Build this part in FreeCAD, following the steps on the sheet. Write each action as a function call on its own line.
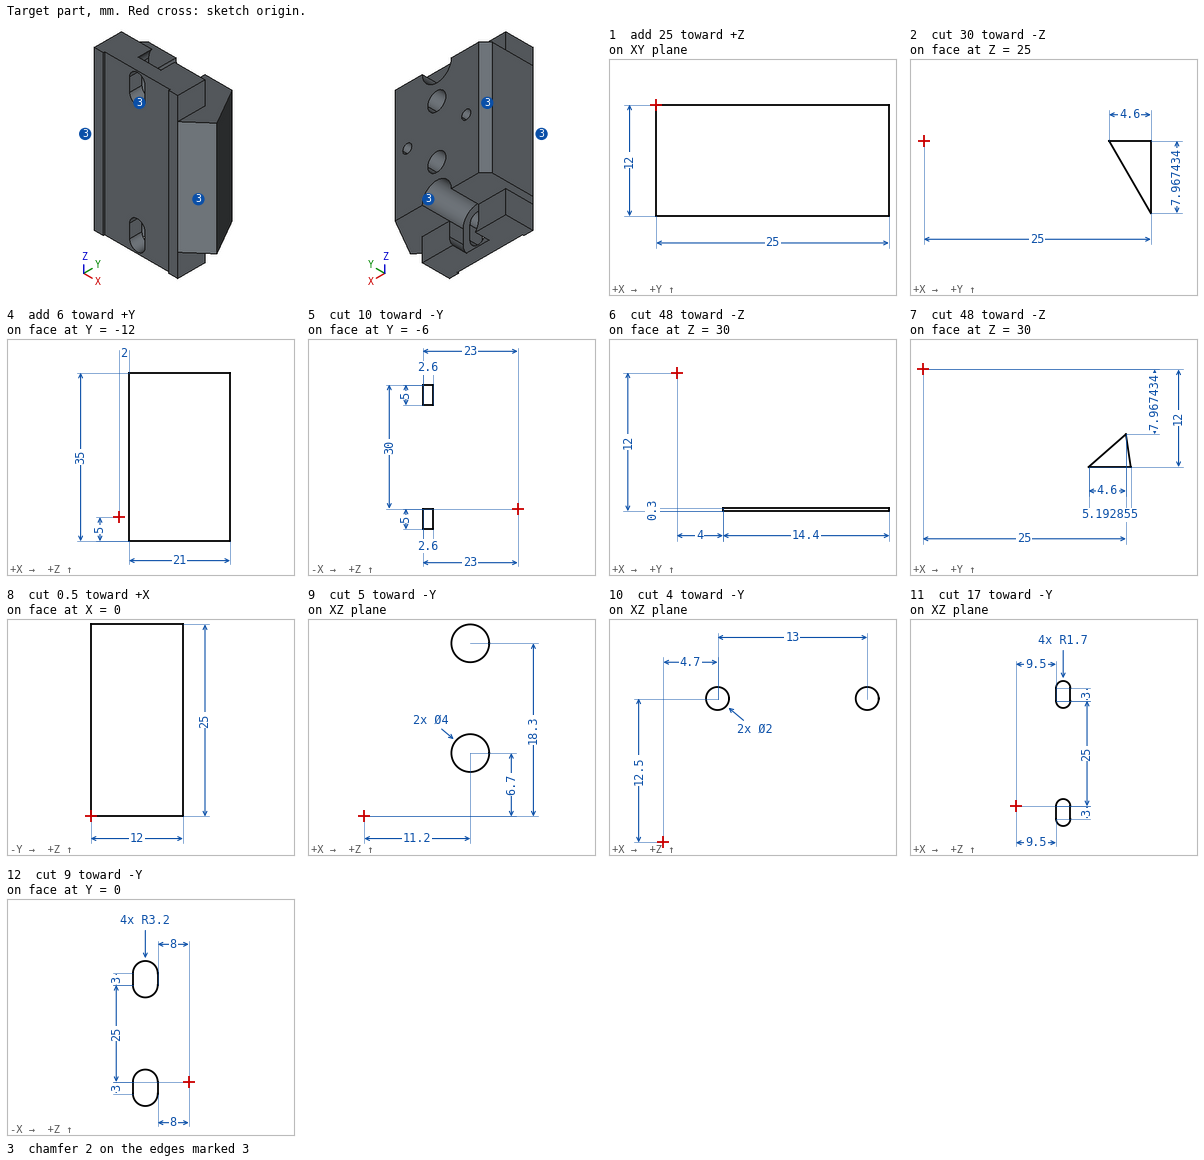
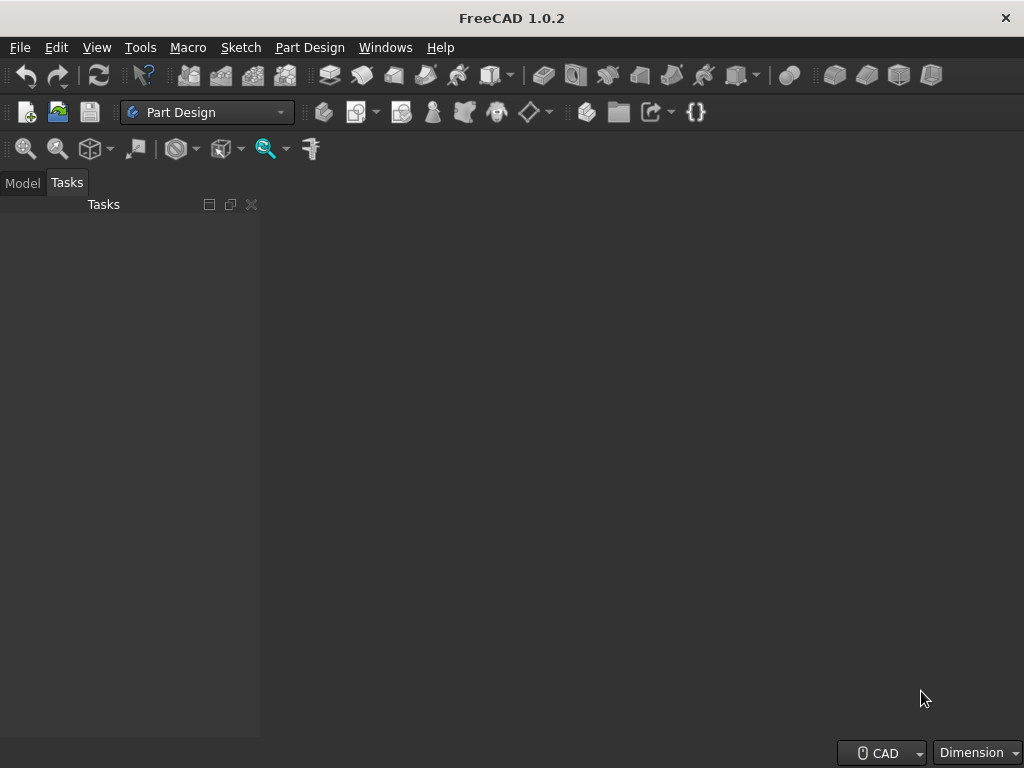
key(ctrl+n)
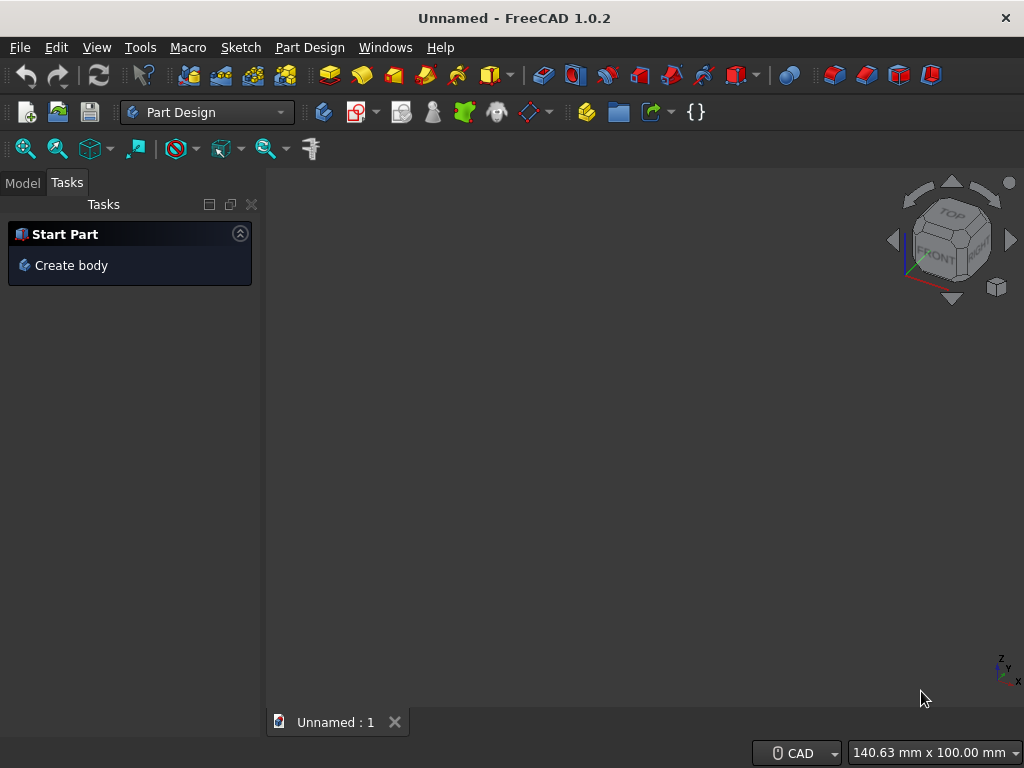
click(356, 112)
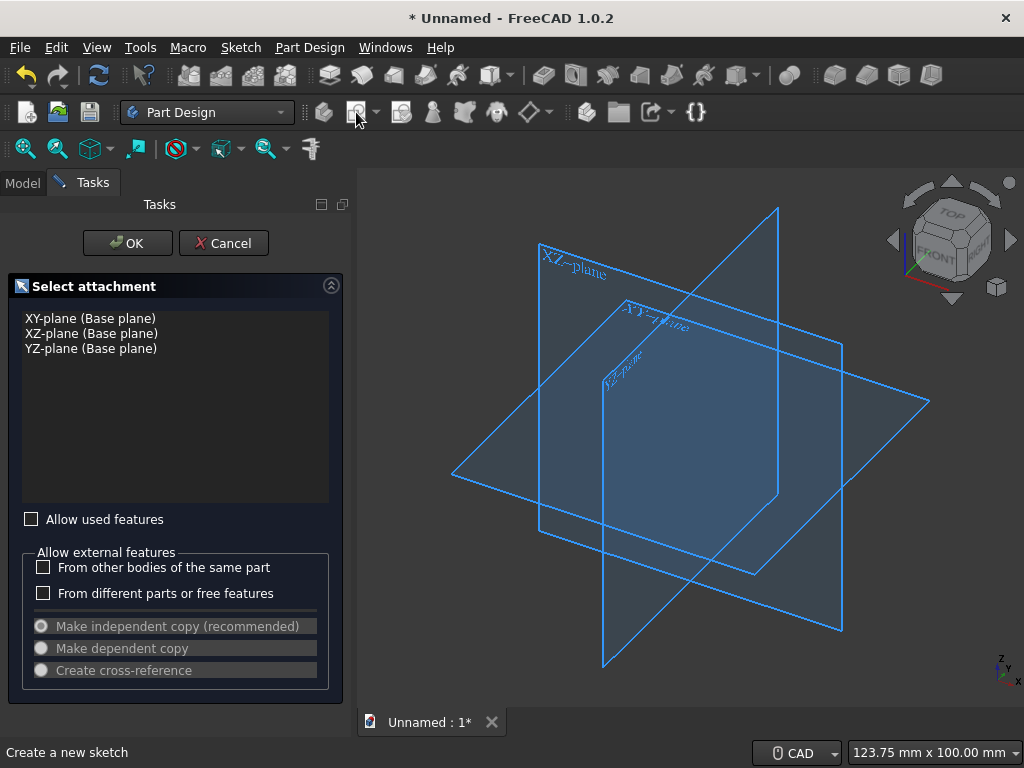
click(82, 318)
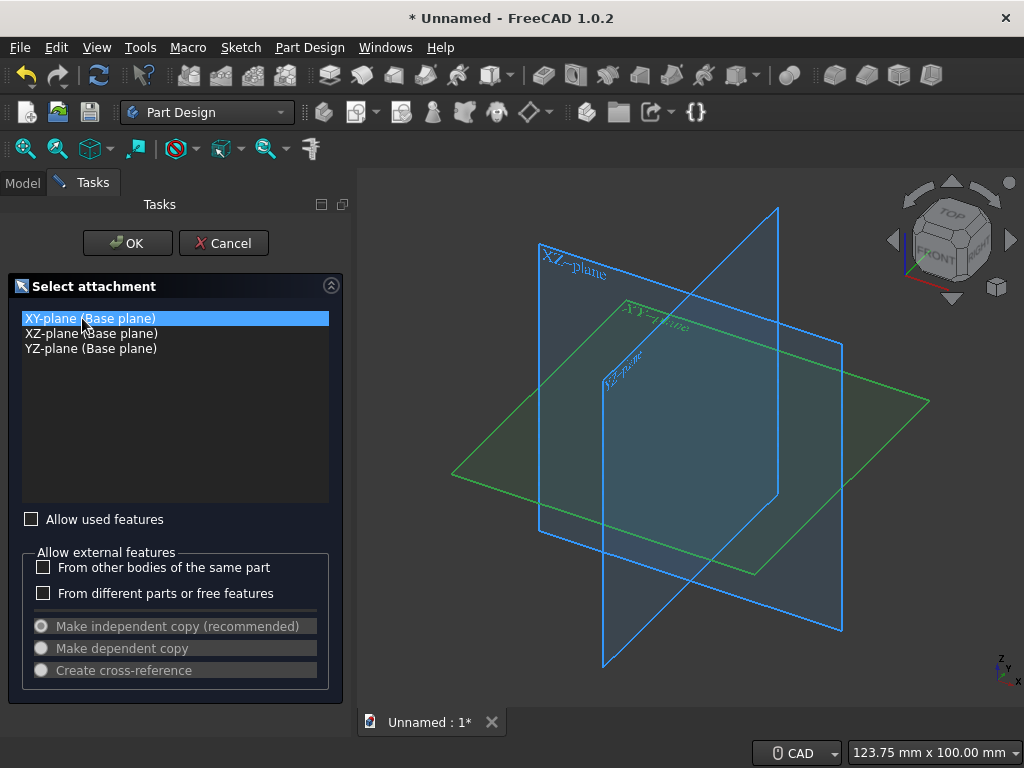
click(128, 243)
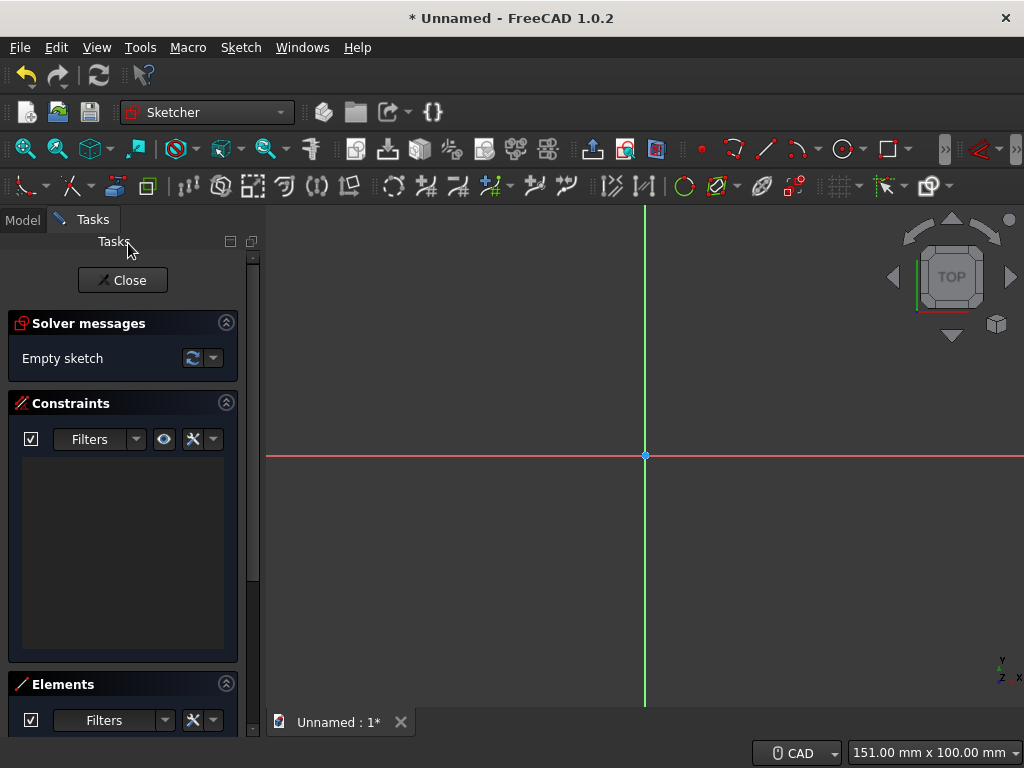
scroll(764, 499, up, 6)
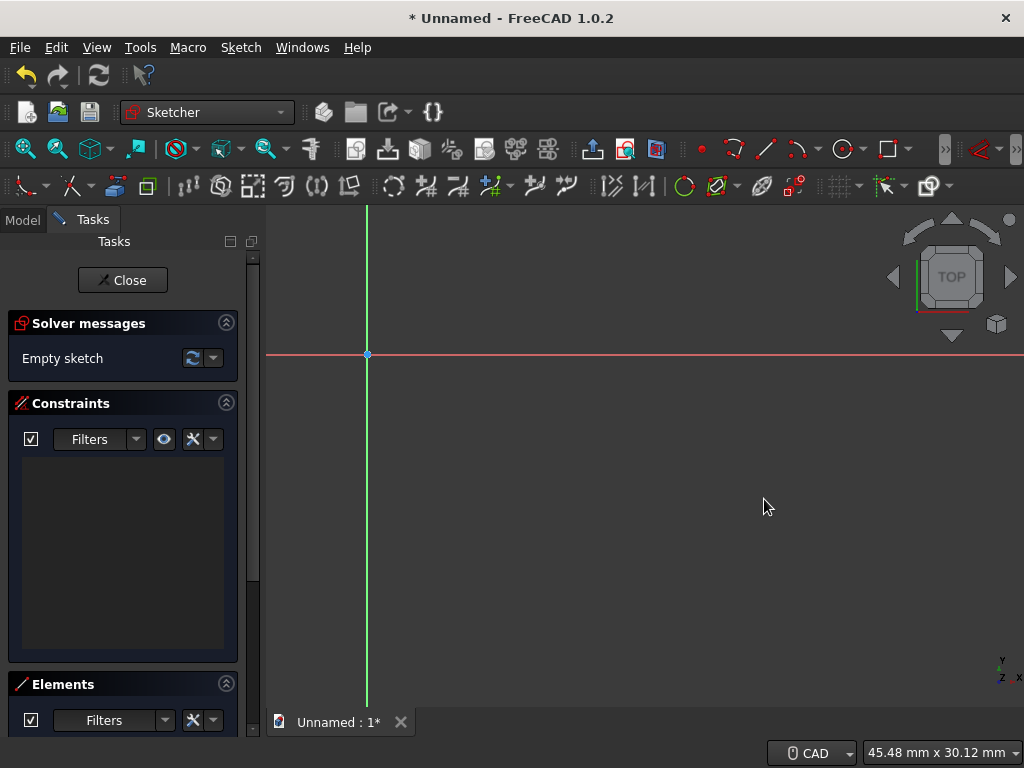
click(888, 150)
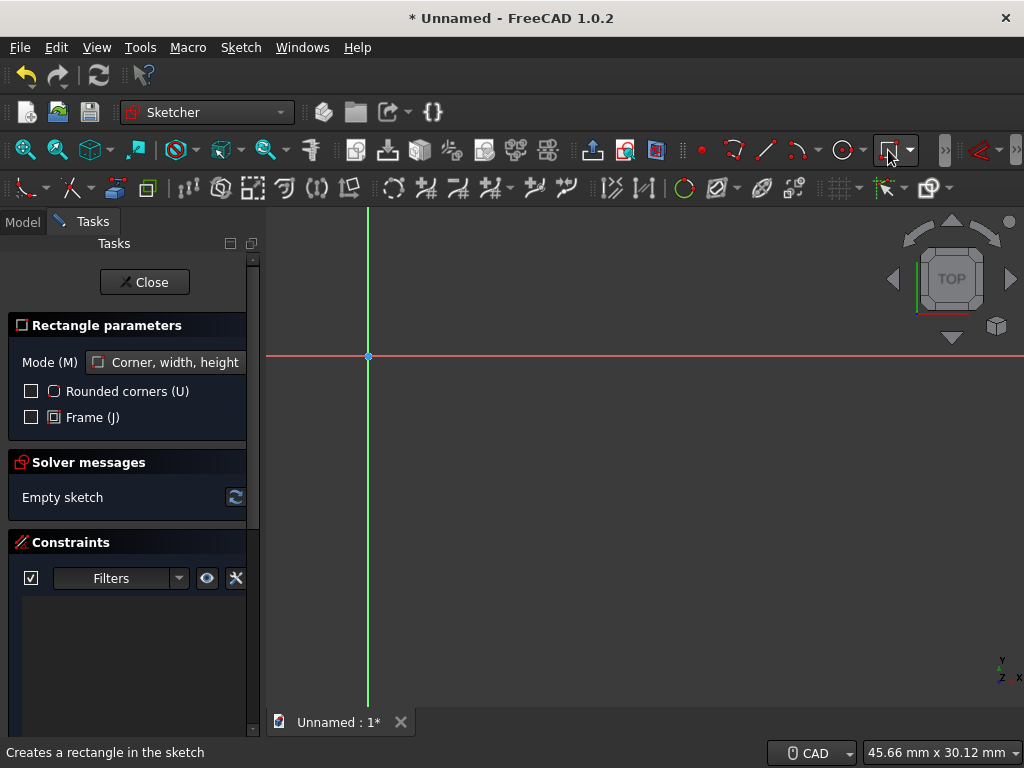
click(368, 356)
click(784, 555)
key(Escape)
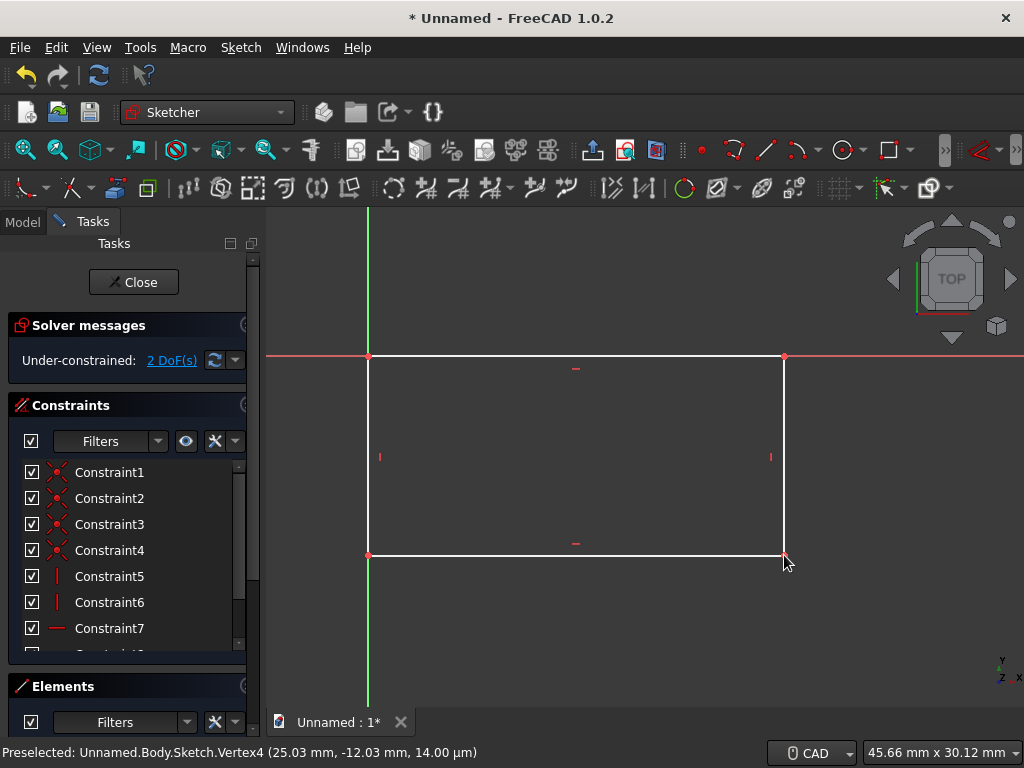
click(368, 416)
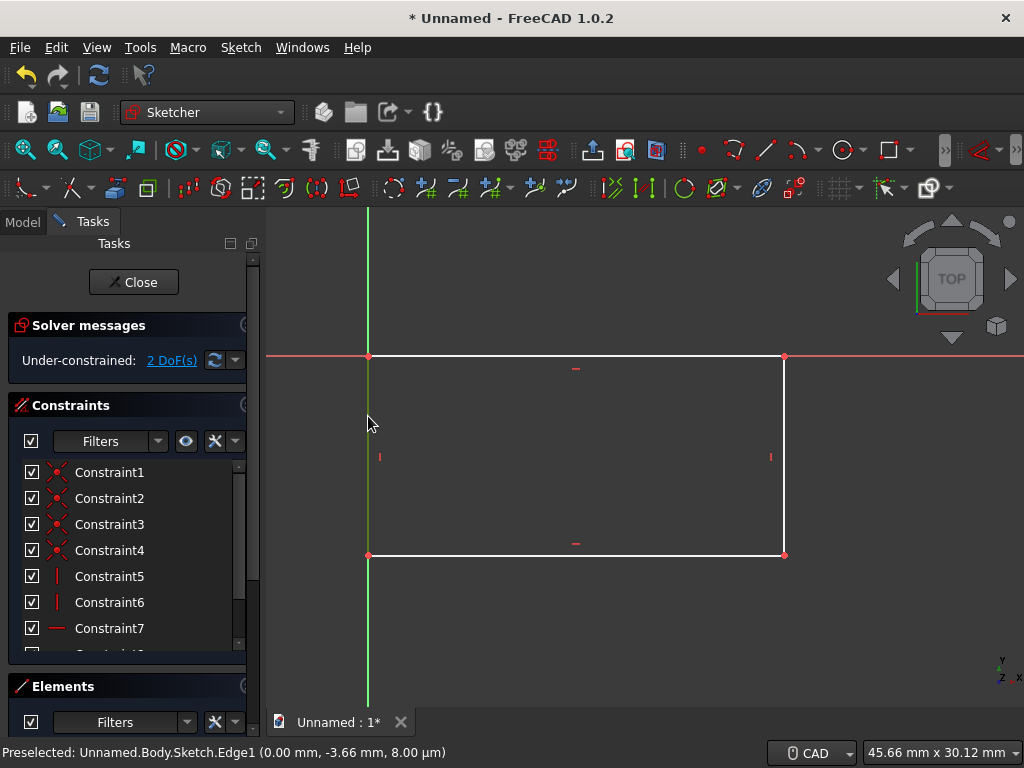
click(1002, 150)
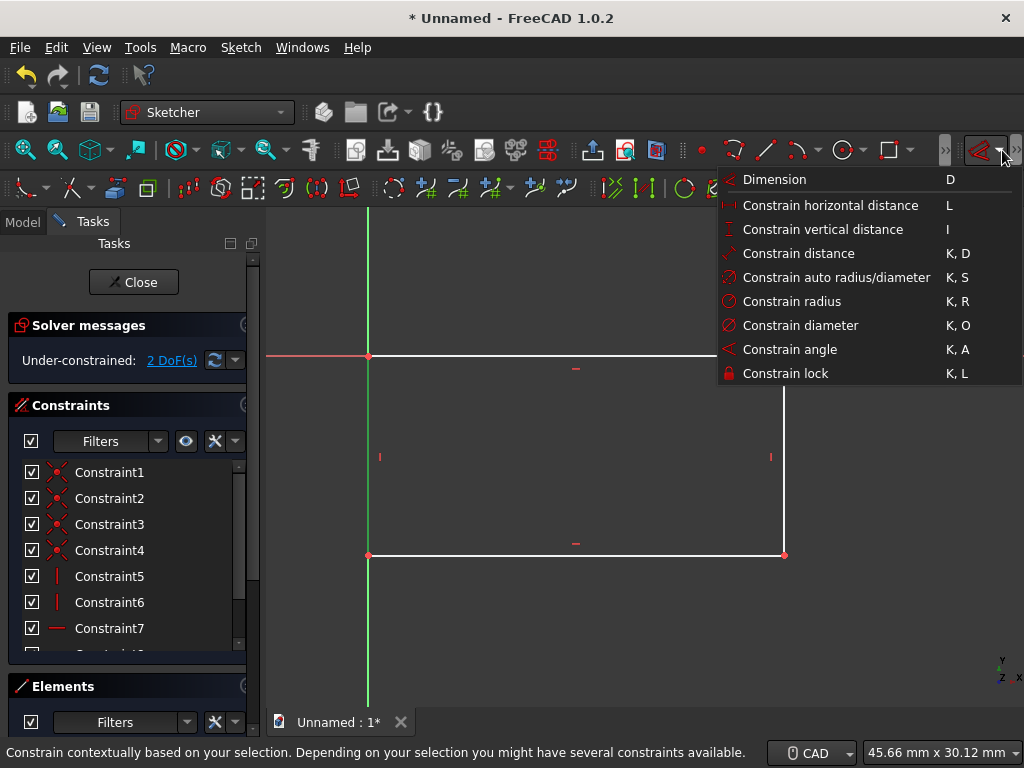
click(870, 229)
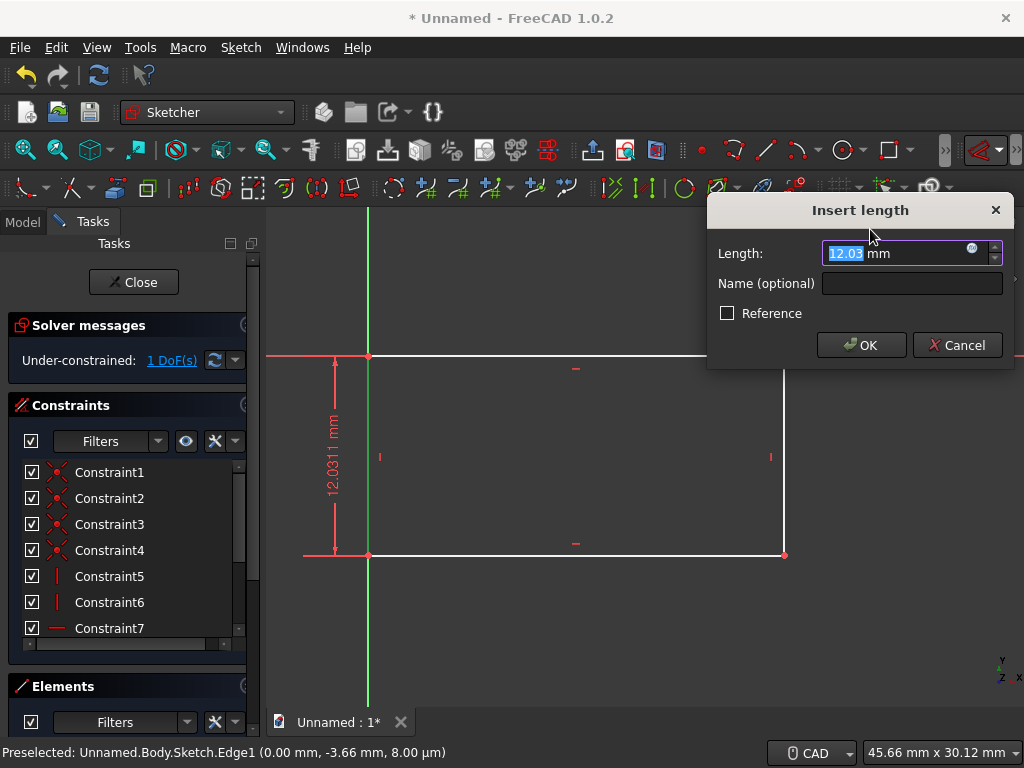
text(12)
key(Return)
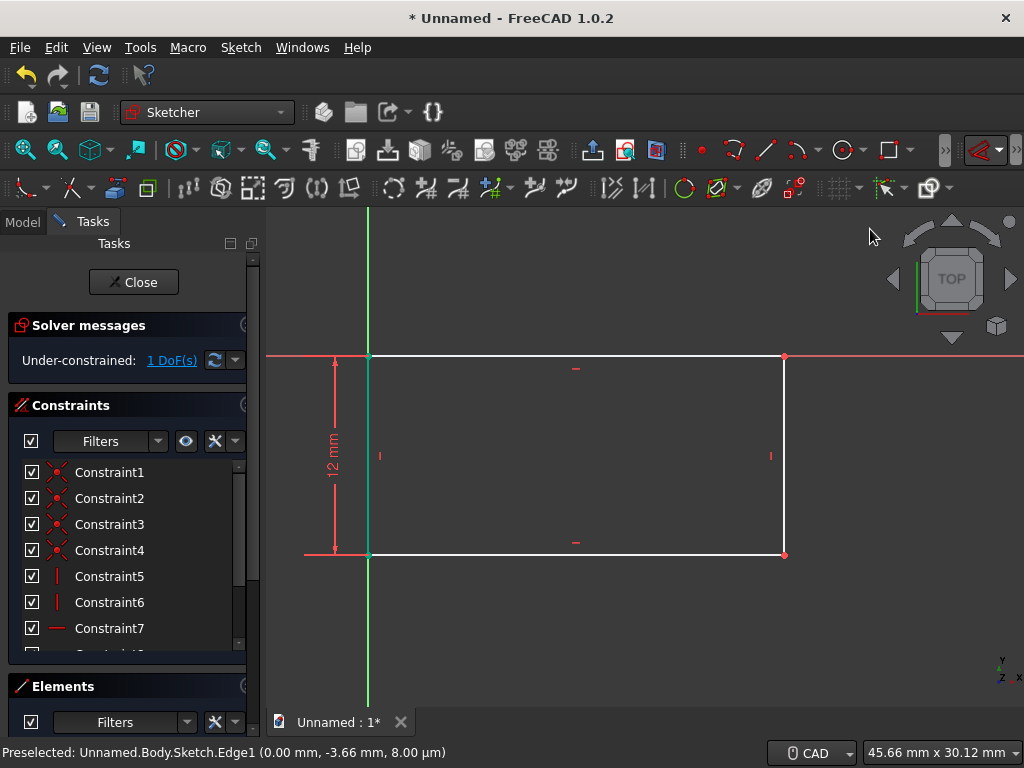
click(493, 555)